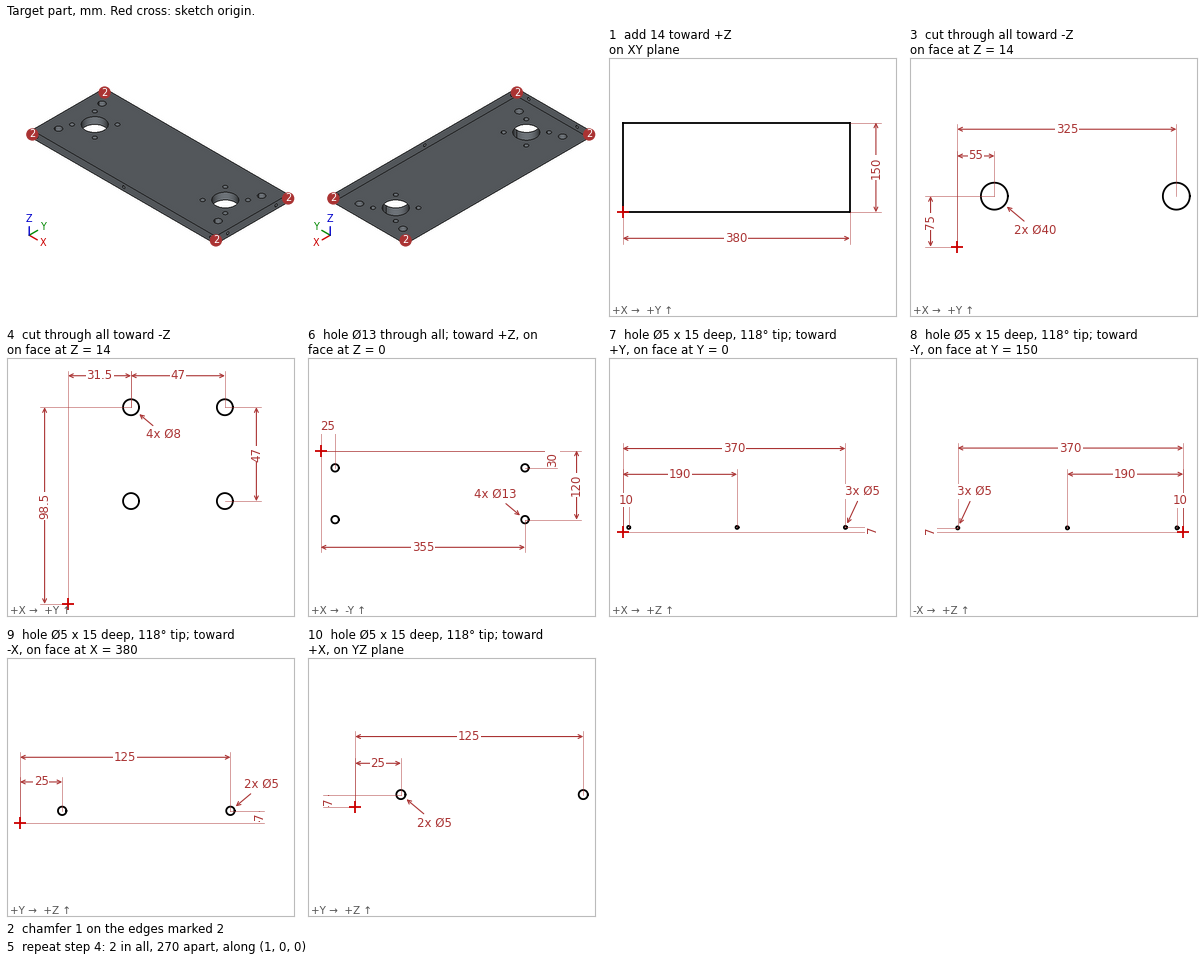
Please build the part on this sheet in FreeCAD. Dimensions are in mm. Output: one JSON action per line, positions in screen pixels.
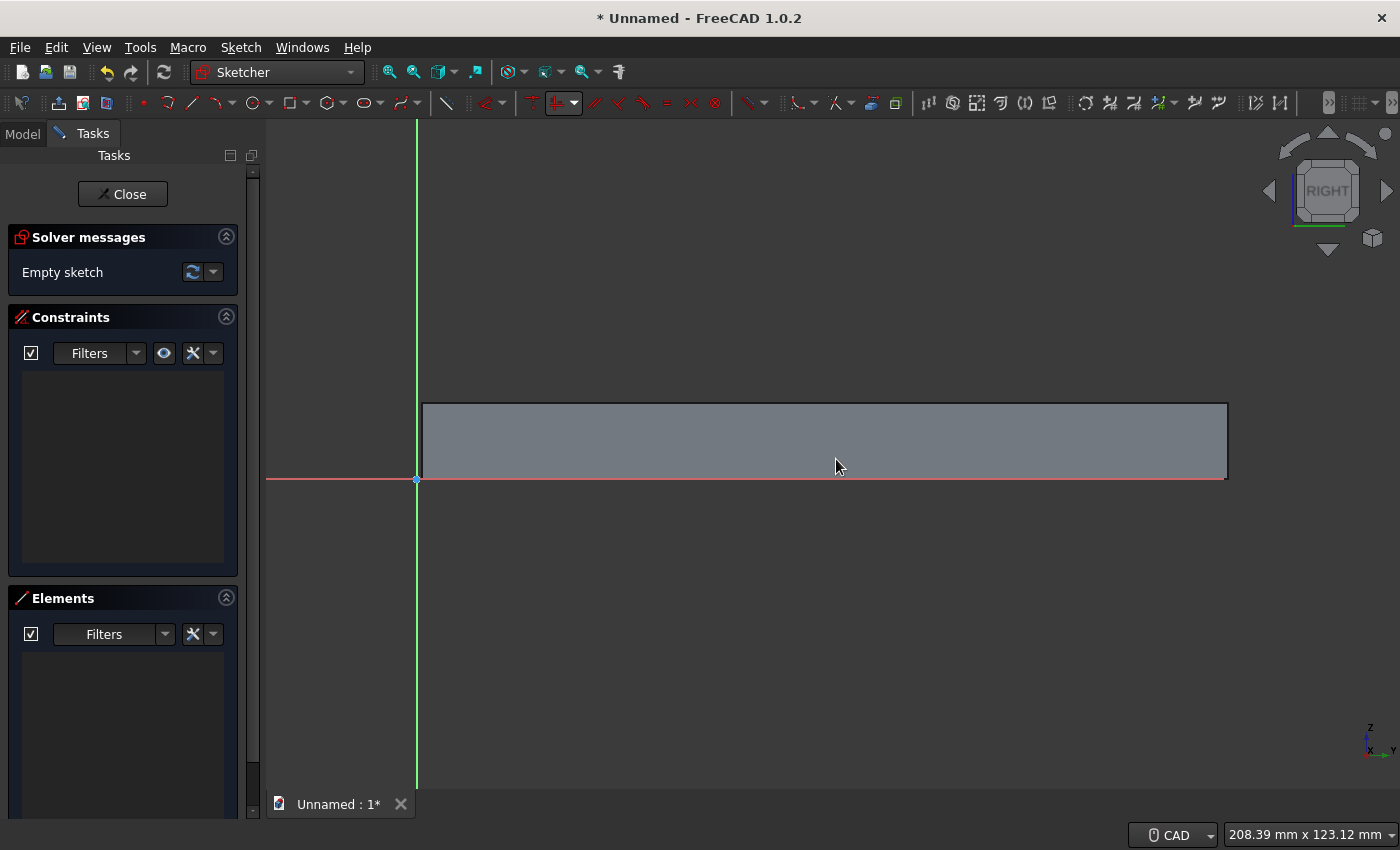
{"action": "left_click", "coordinate": [254, 104]}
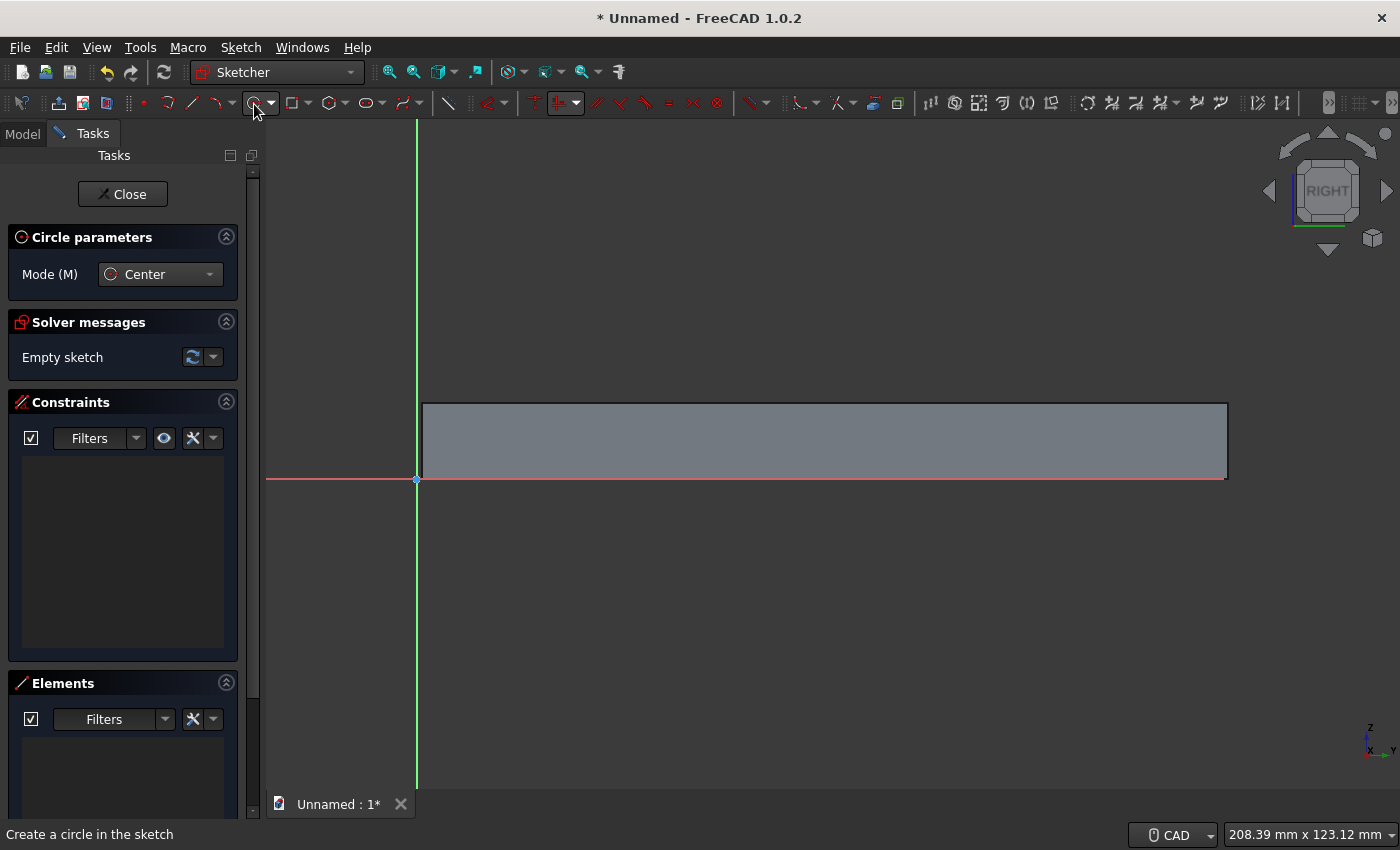
{"action": "scroll", "coordinate": [553, 441], "scroll_direction": "up", "scroll_amount": 3}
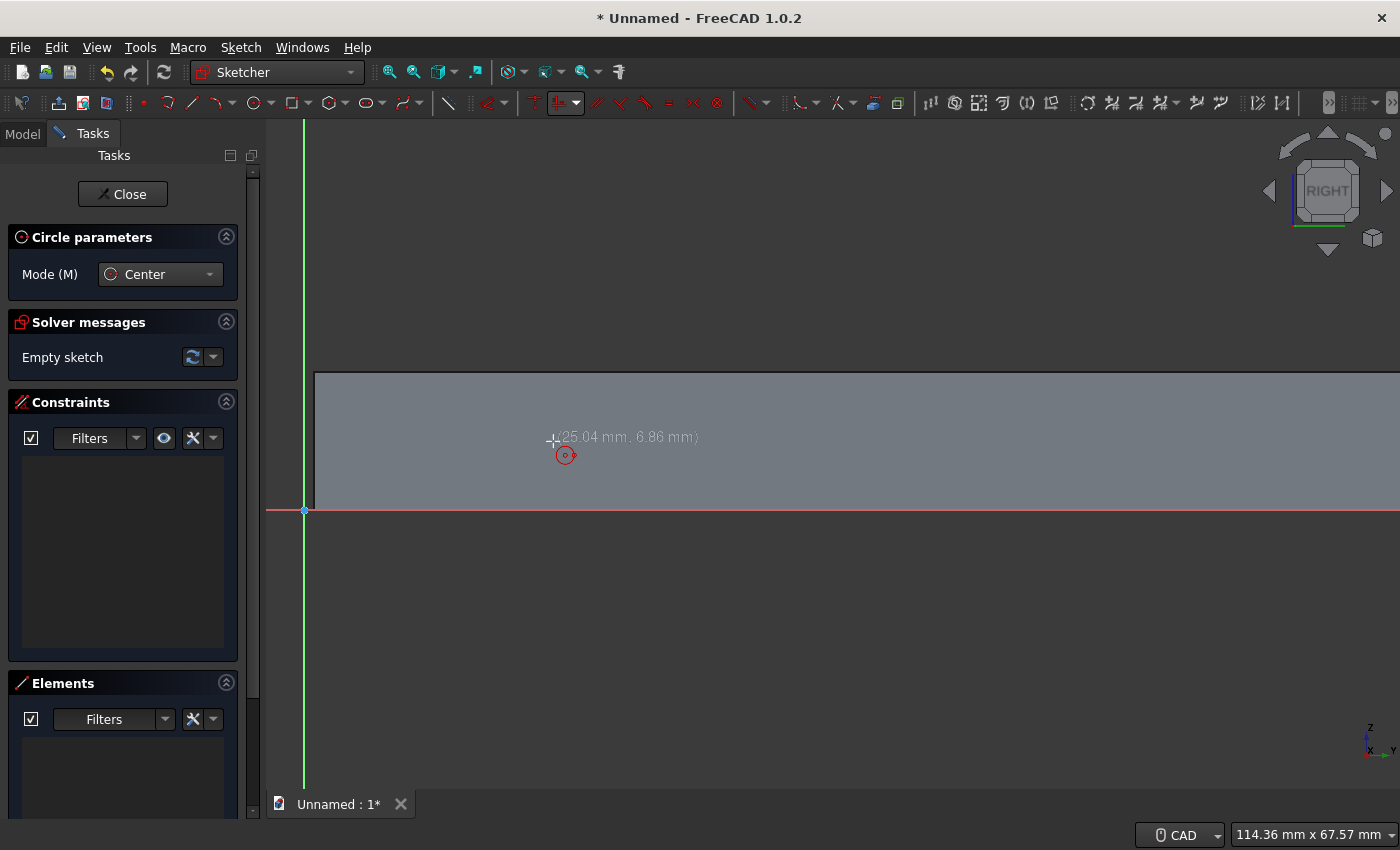
{"action": "left_click", "coordinate": [552, 441]}
{"action": "mouse_move", "coordinate": [570, 423]}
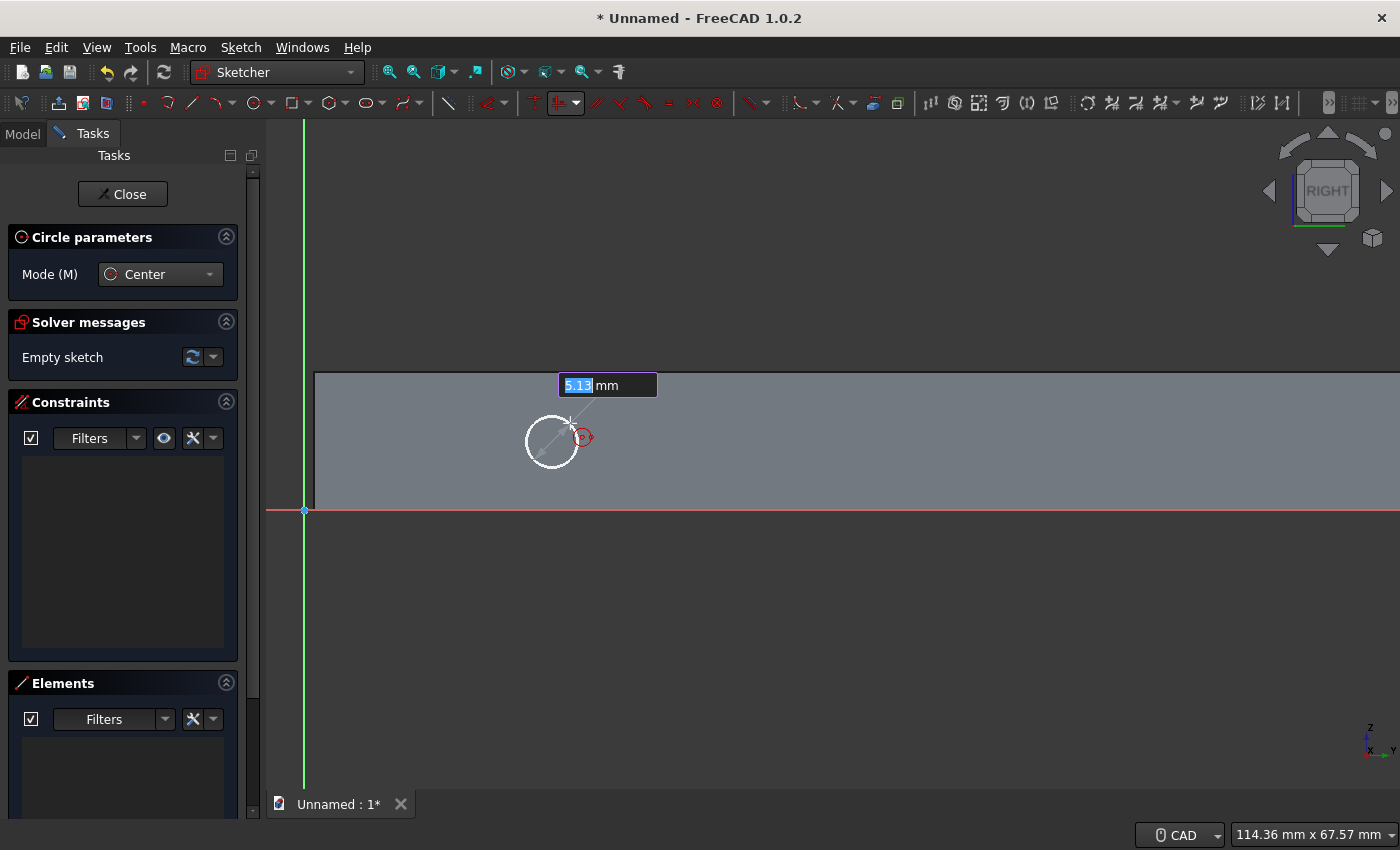
{"action": "type", "text": "5"}
{"action": "key", "text": "Return"}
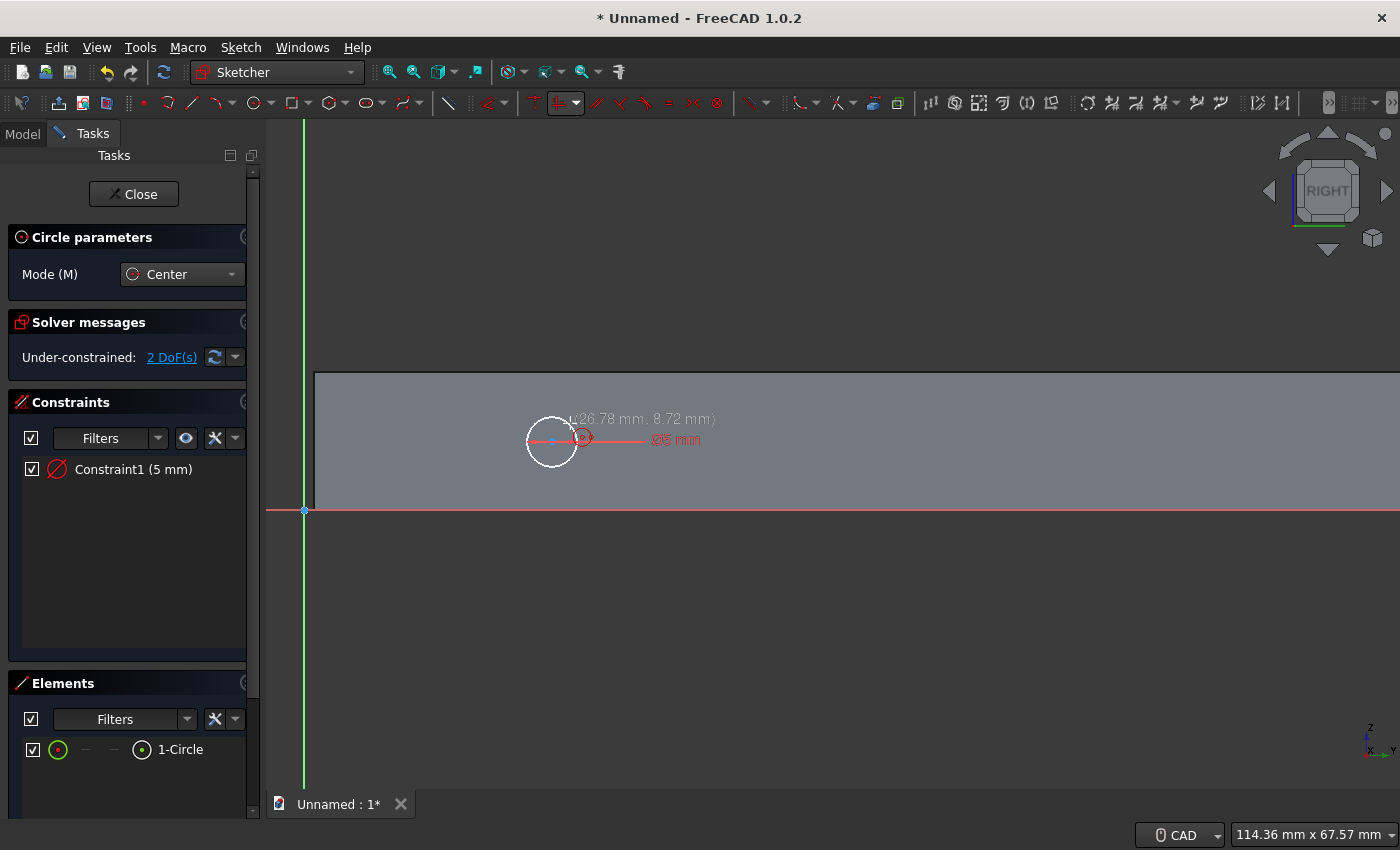
{"action": "scroll", "coordinate": [555, 443], "scroll_direction": "down", "scroll_amount": 3}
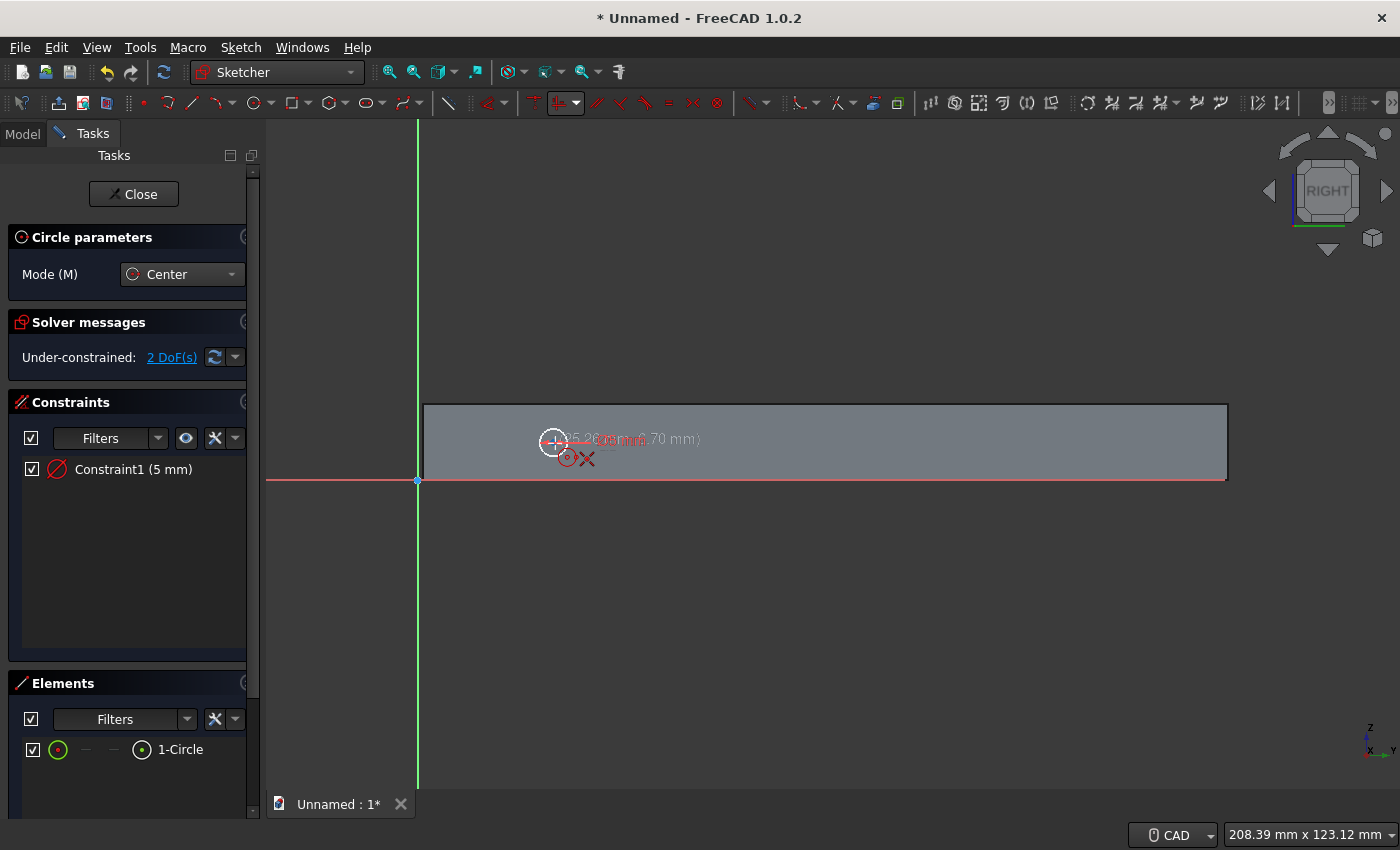
{"action": "scroll", "coordinate": [1098, 442], "scroll_direction": "up", "scroll_amount": 3}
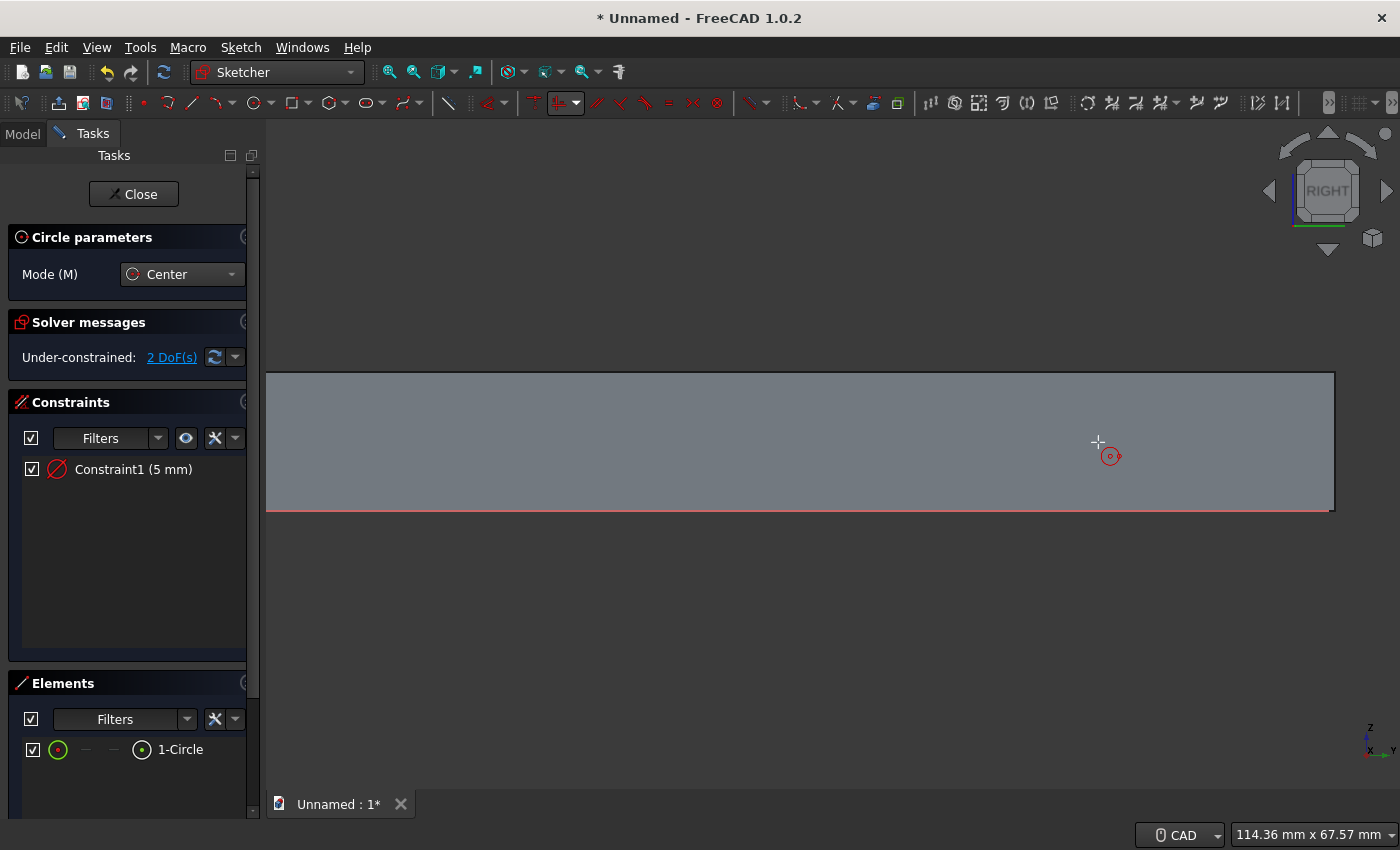
{"action": "left_click", "coordinate": [1097, 442]}
{"action": "mouse_move", "coordinate": [1115, 424]}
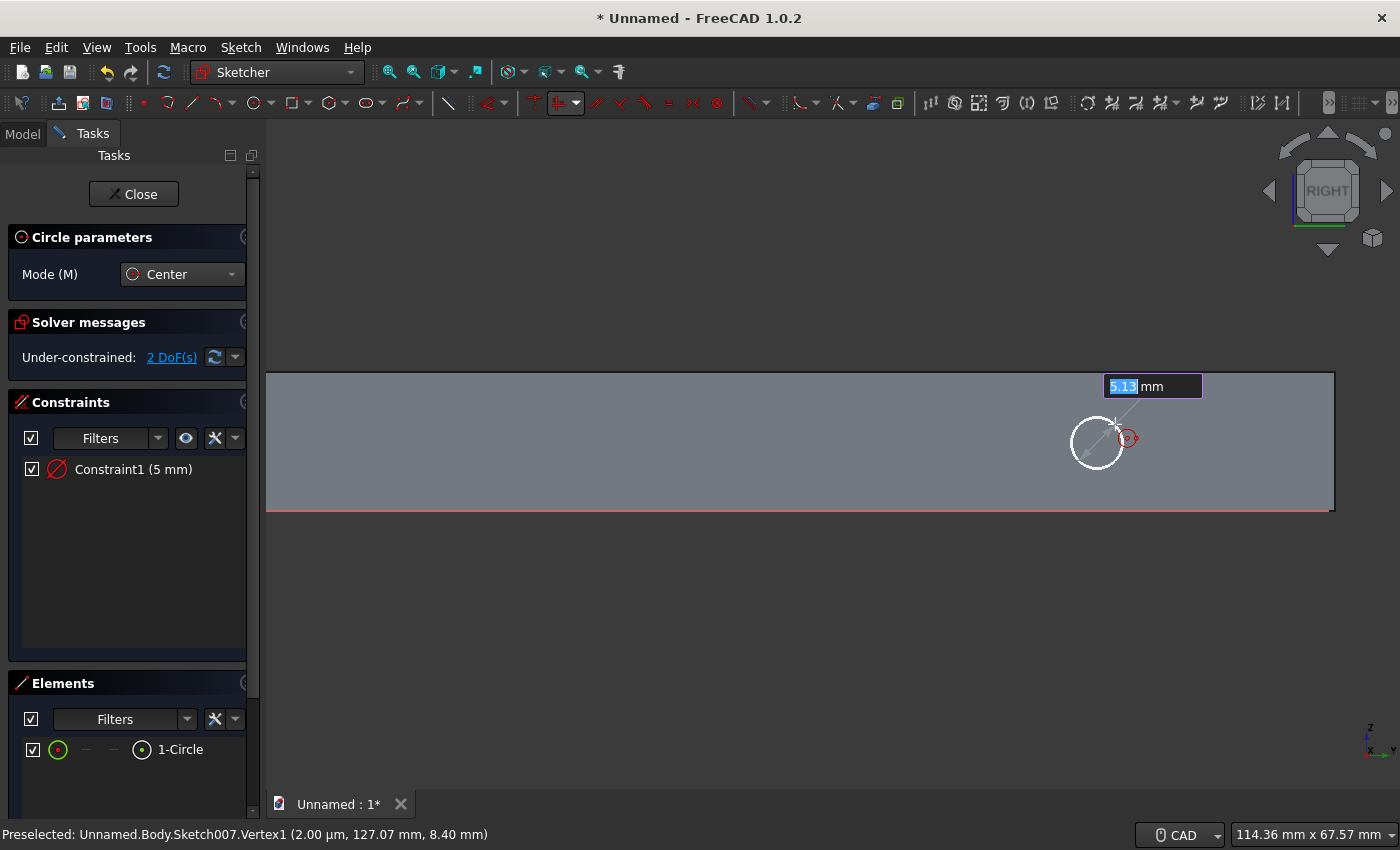
{"action": "type", "text": "5"}
{"action": "key", "text": "Return"}
{"action": "key", "text": "Escape"}